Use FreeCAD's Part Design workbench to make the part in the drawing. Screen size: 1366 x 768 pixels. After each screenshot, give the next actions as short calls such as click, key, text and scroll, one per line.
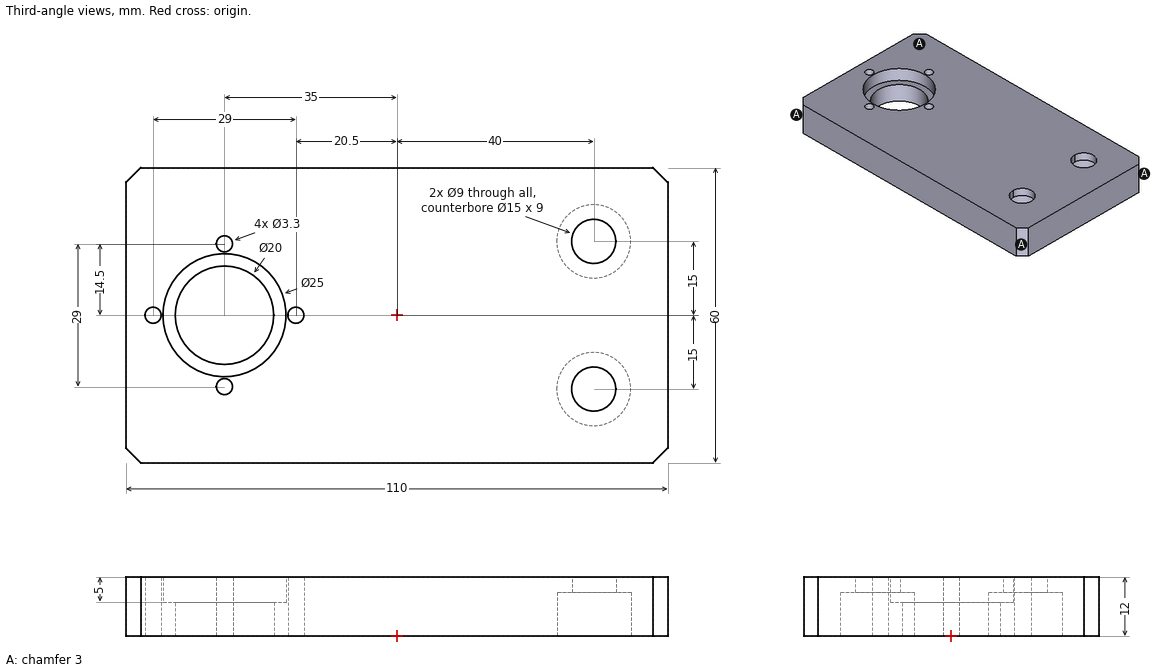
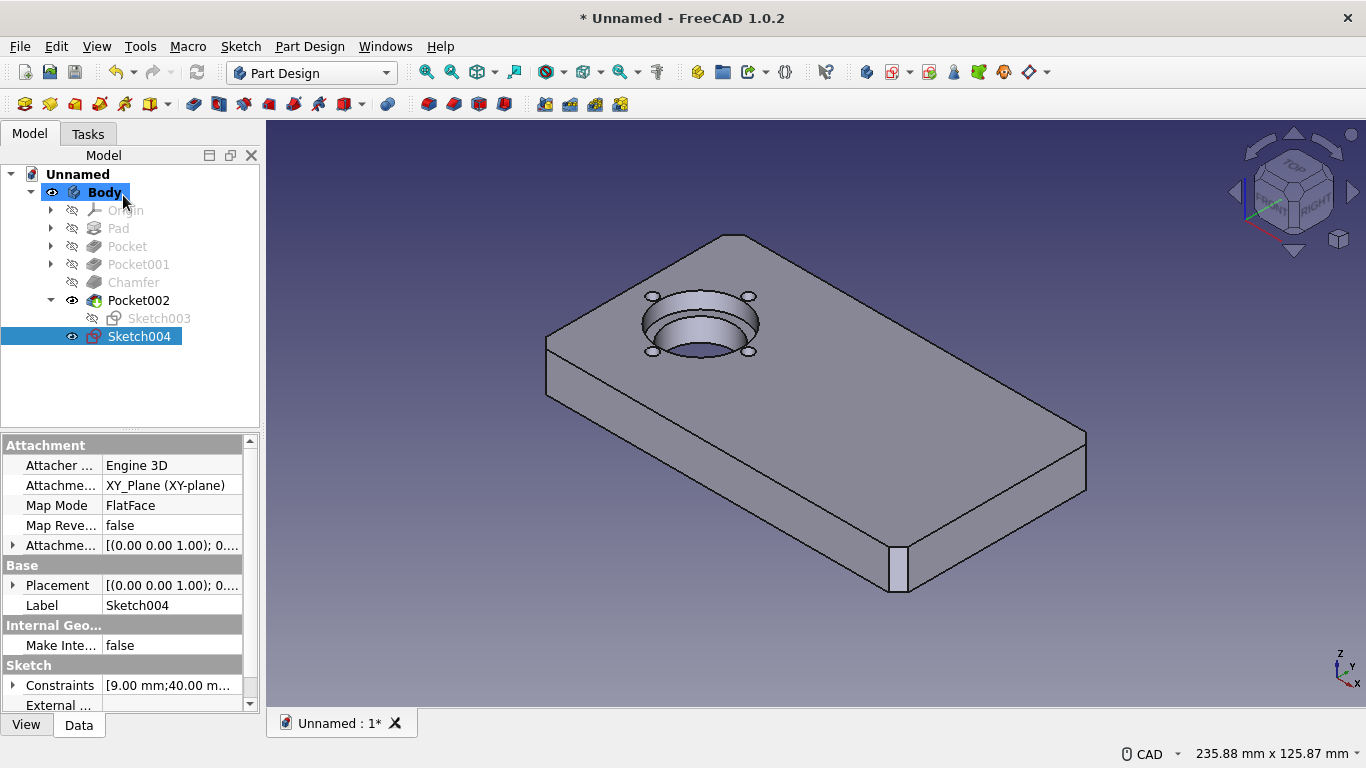
click(219, 104)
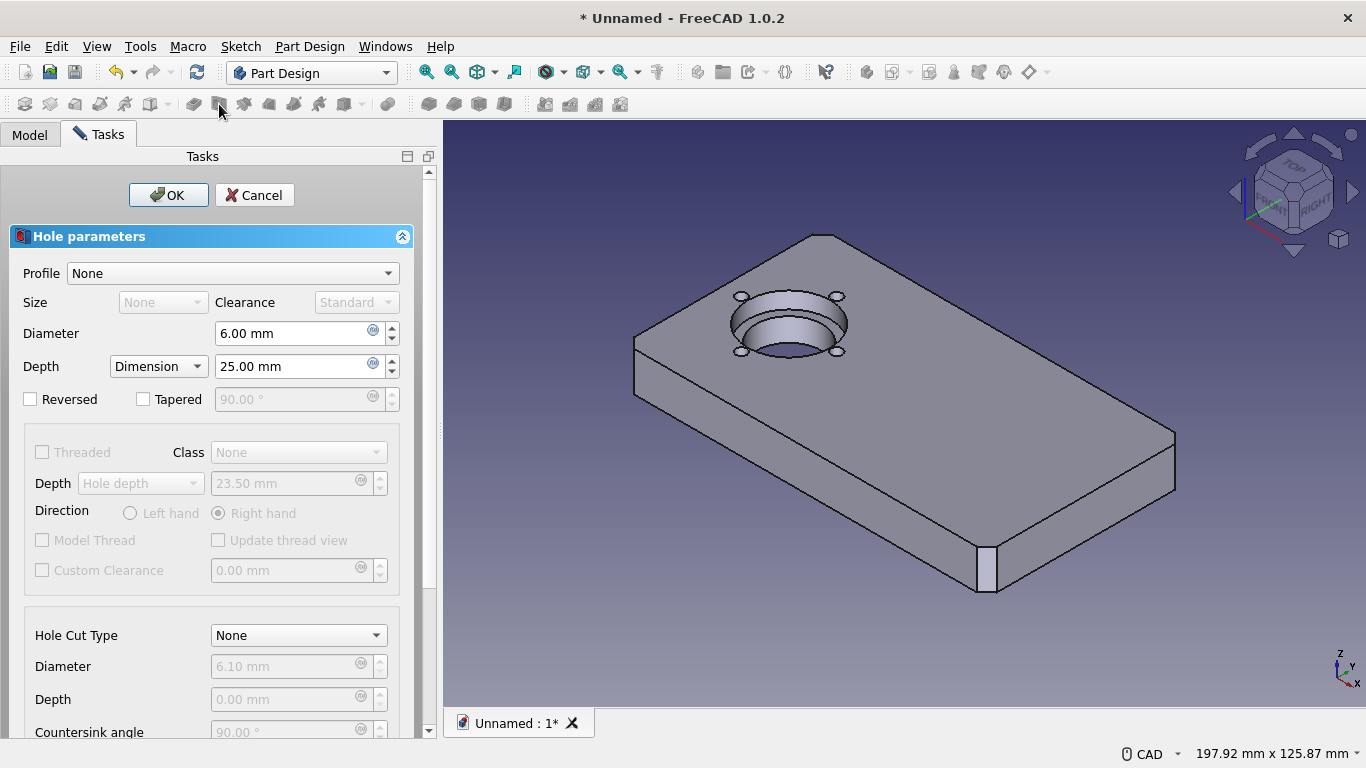
triple_click(300, 334)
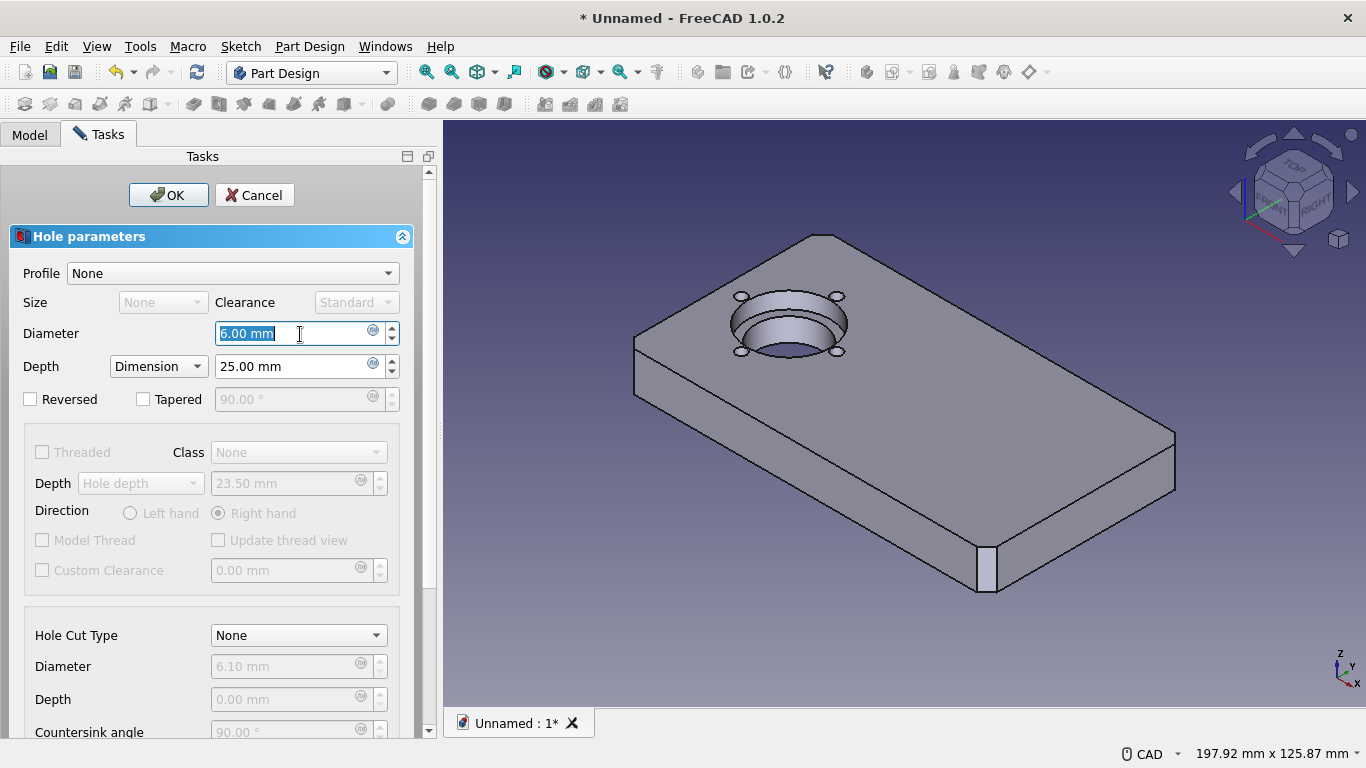
text(9)
key(Tab)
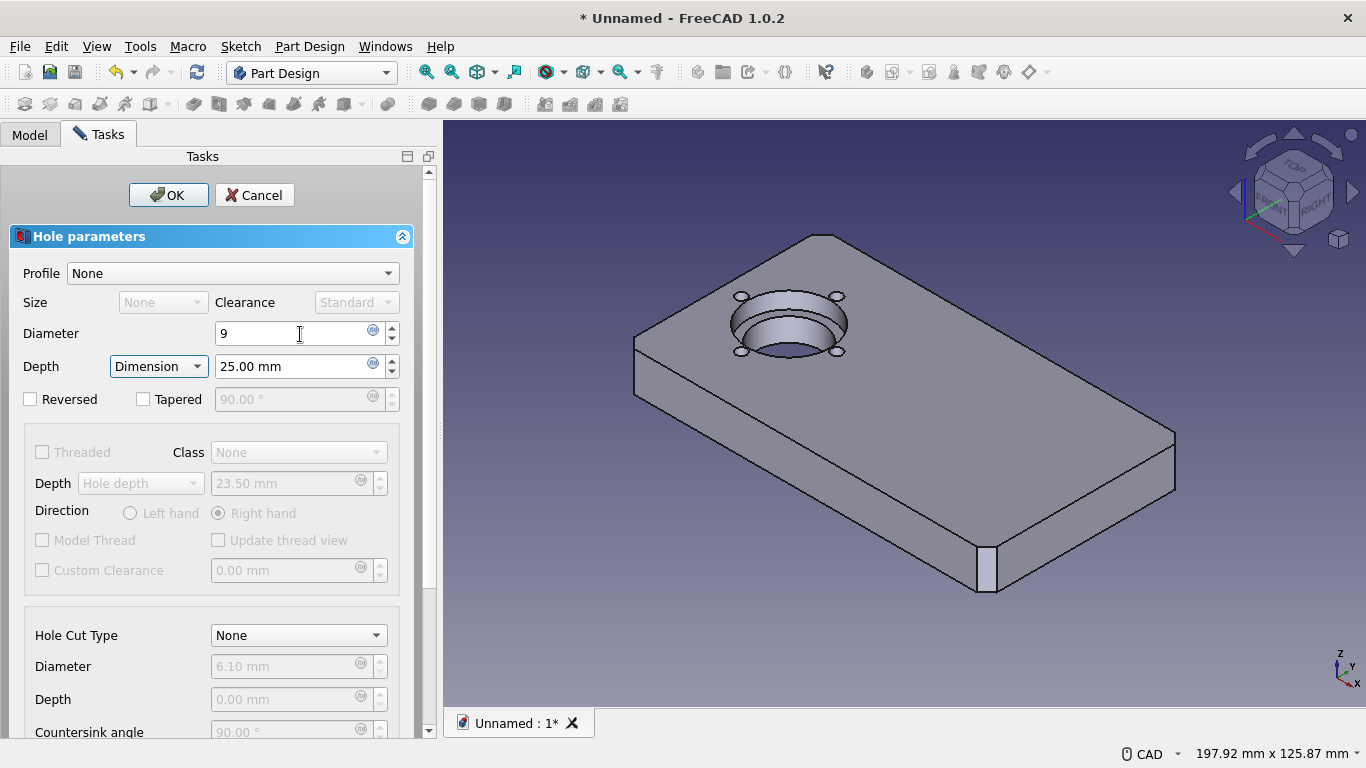
click(160, 366)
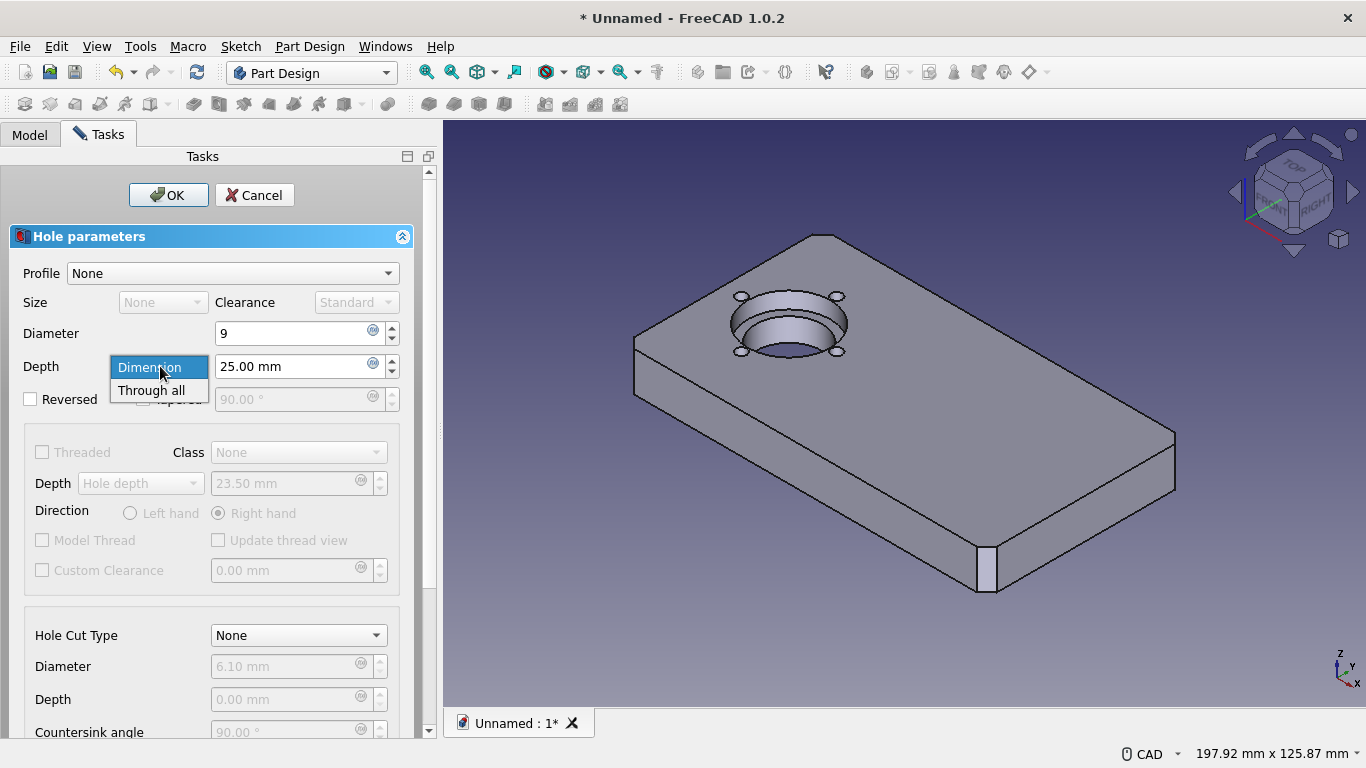
click(158, 390)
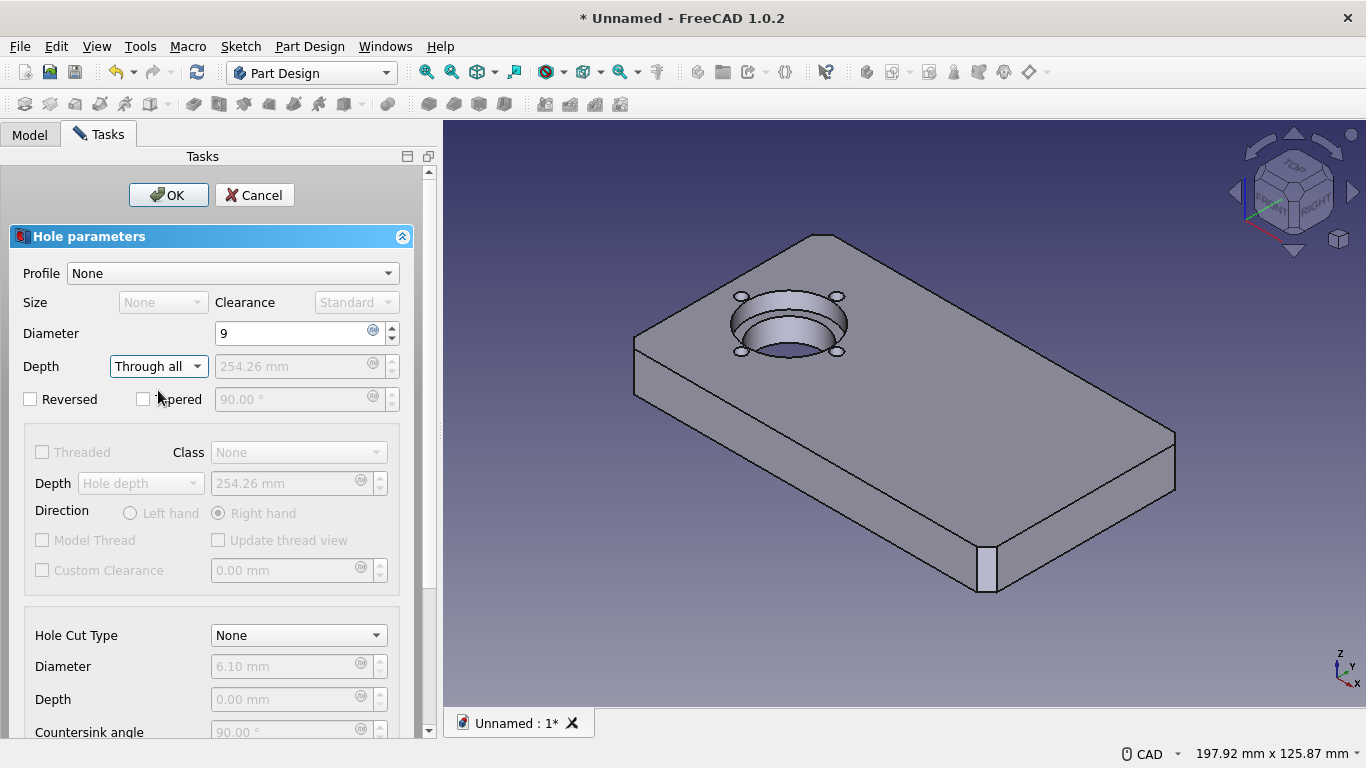
click(31, 399)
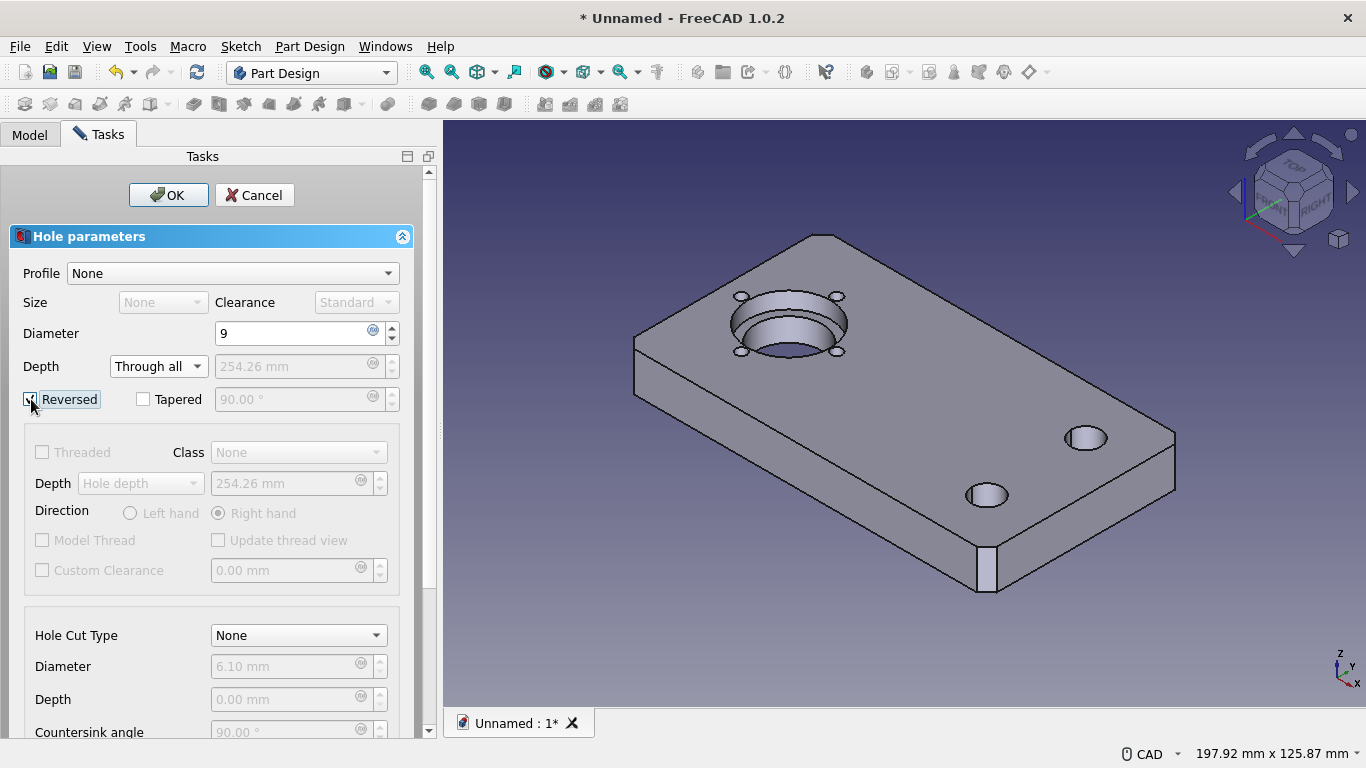
click(300, 636)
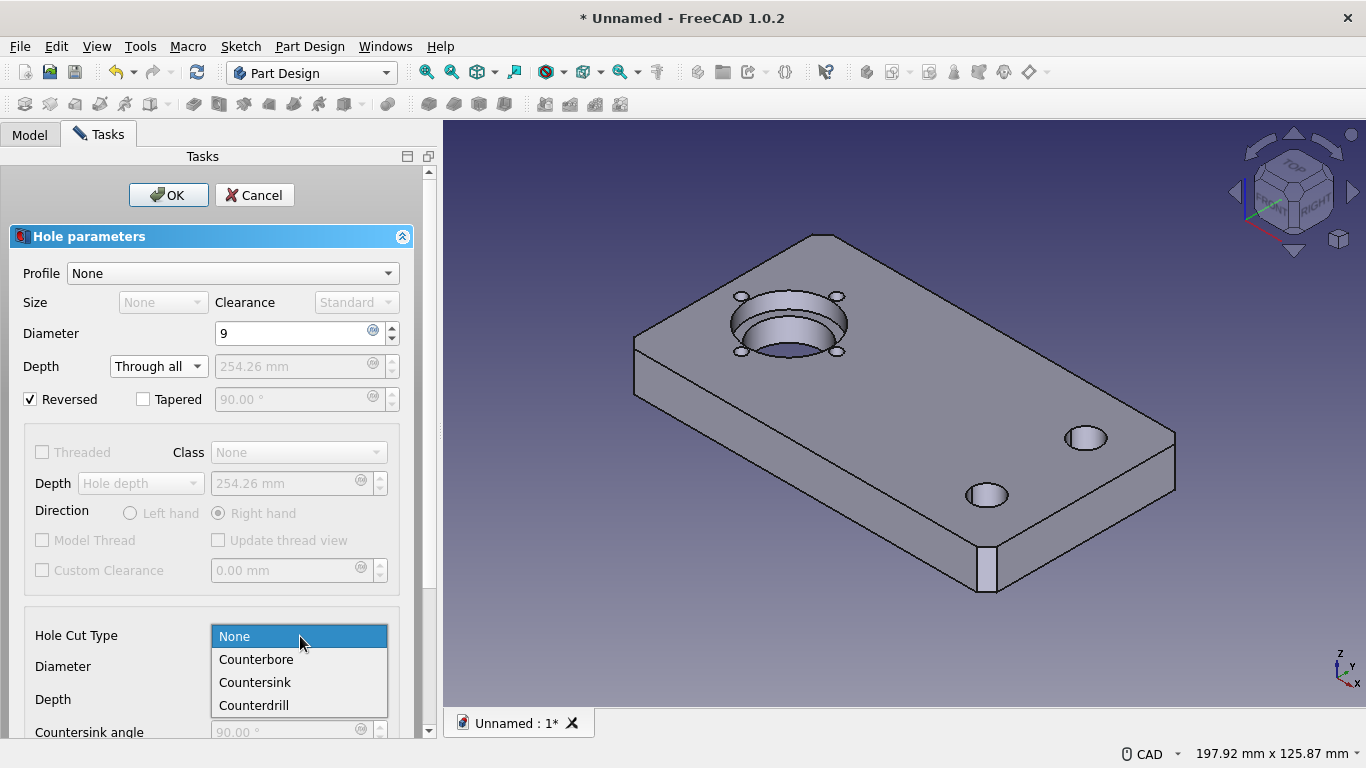
click(298, 660)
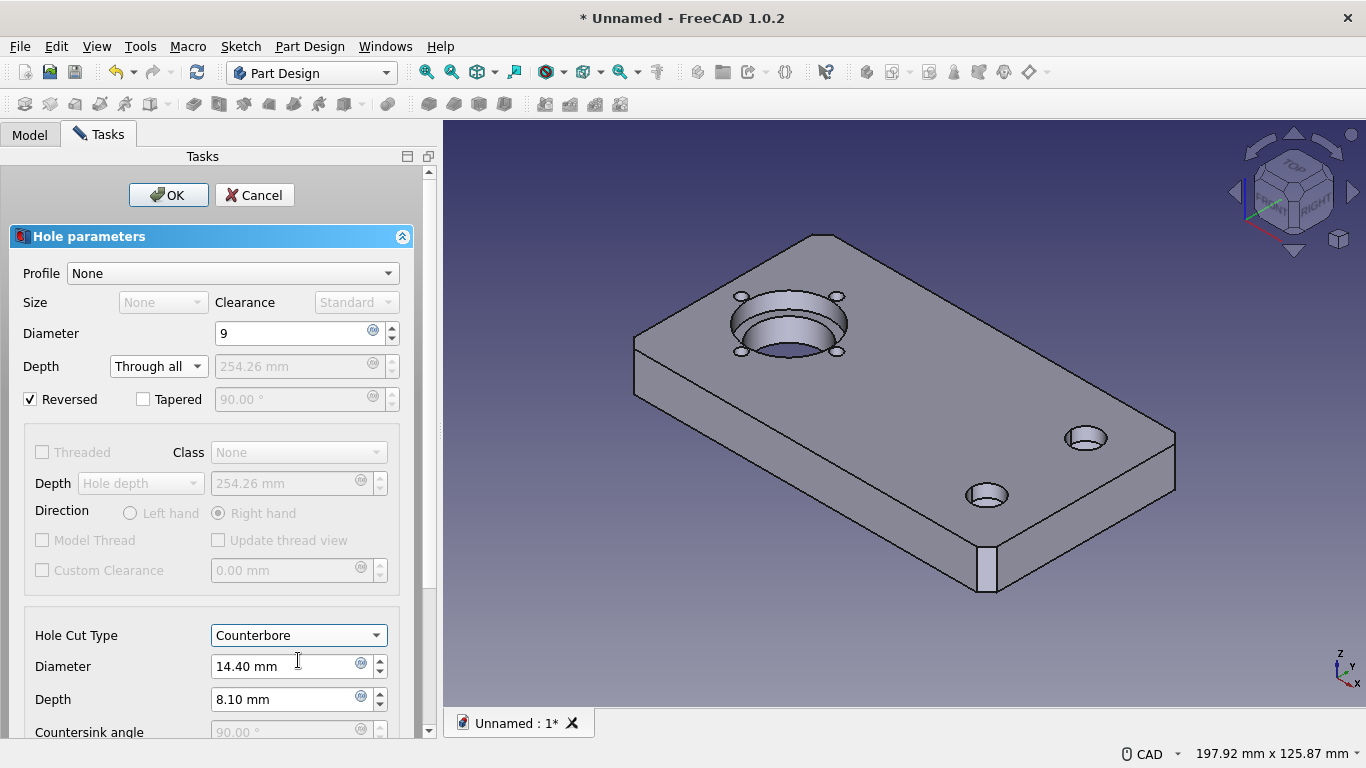
triple_click(292, 666)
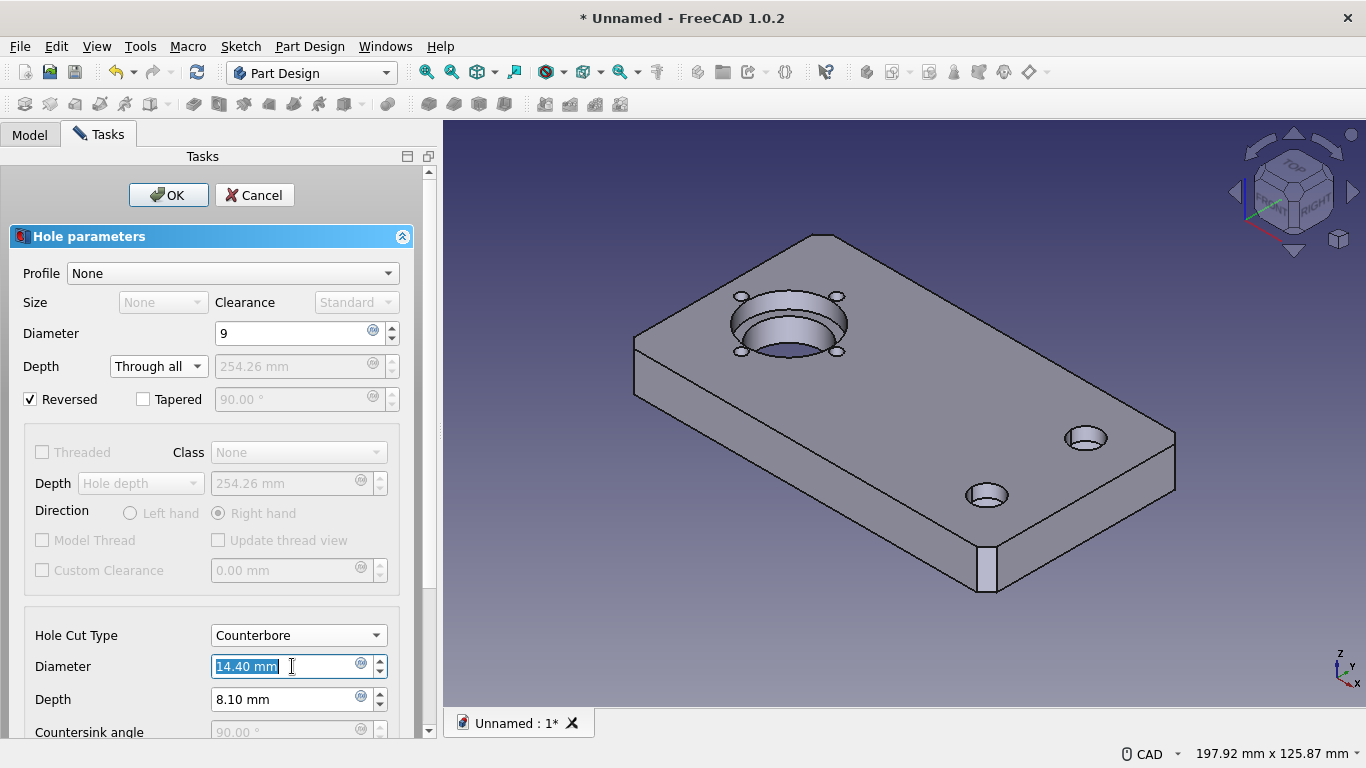
text(15)
key(Tab)